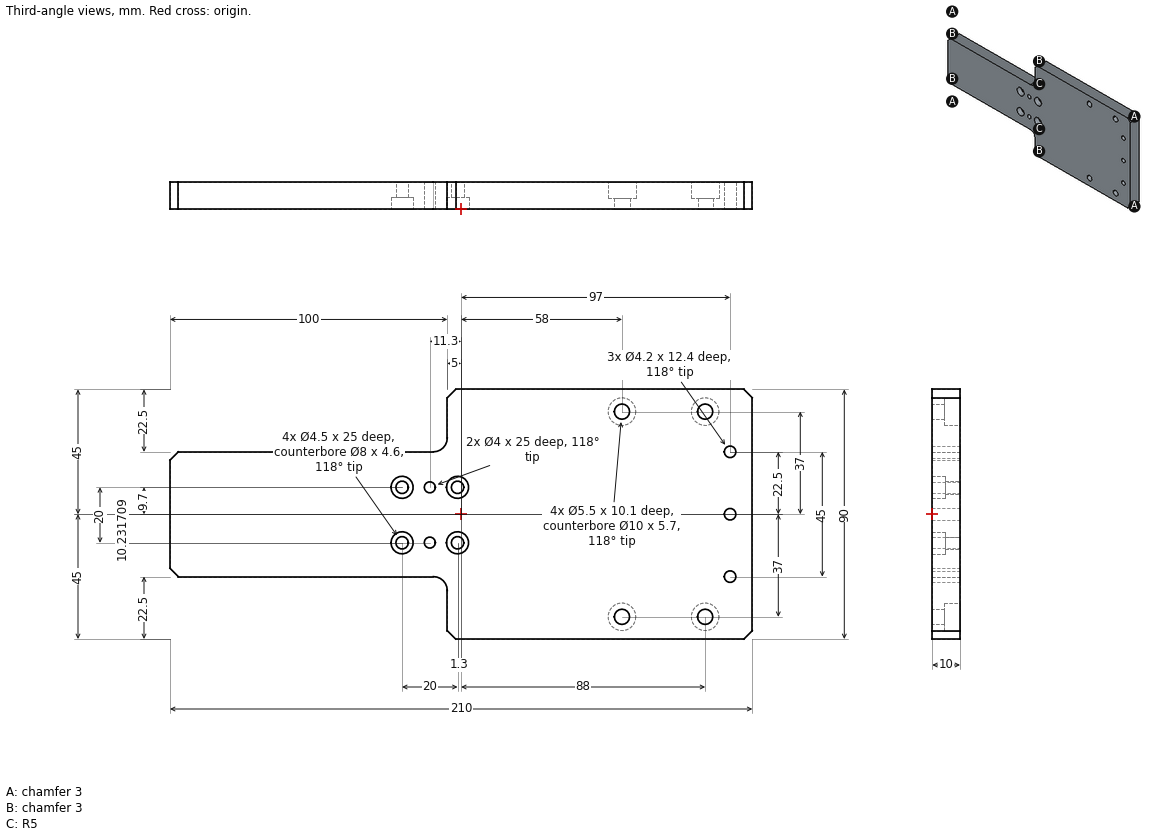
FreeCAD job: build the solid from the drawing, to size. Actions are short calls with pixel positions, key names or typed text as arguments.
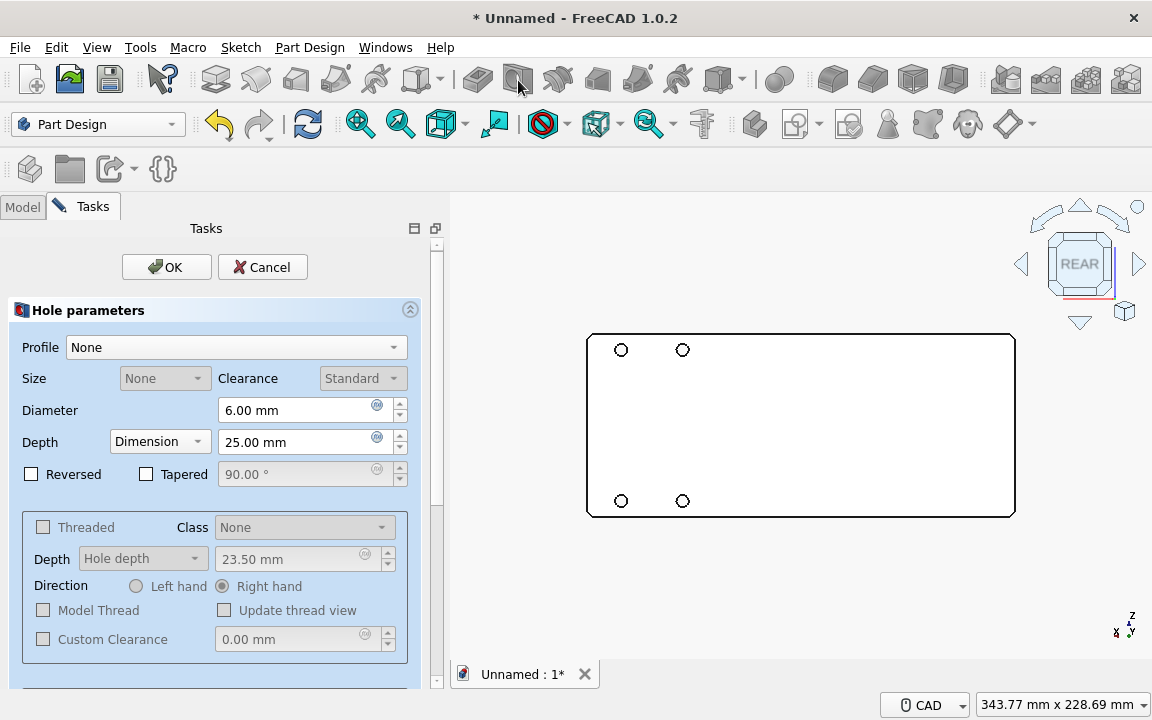
triple_click(305, 410)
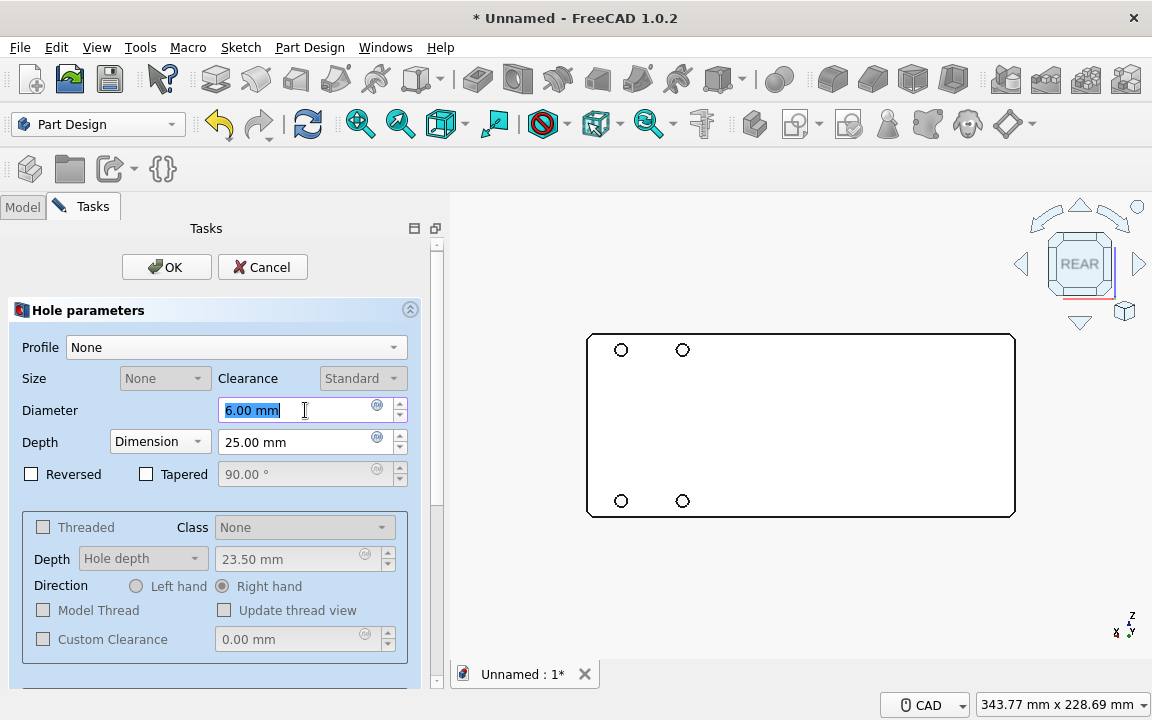
text(5.5)
key(Tab)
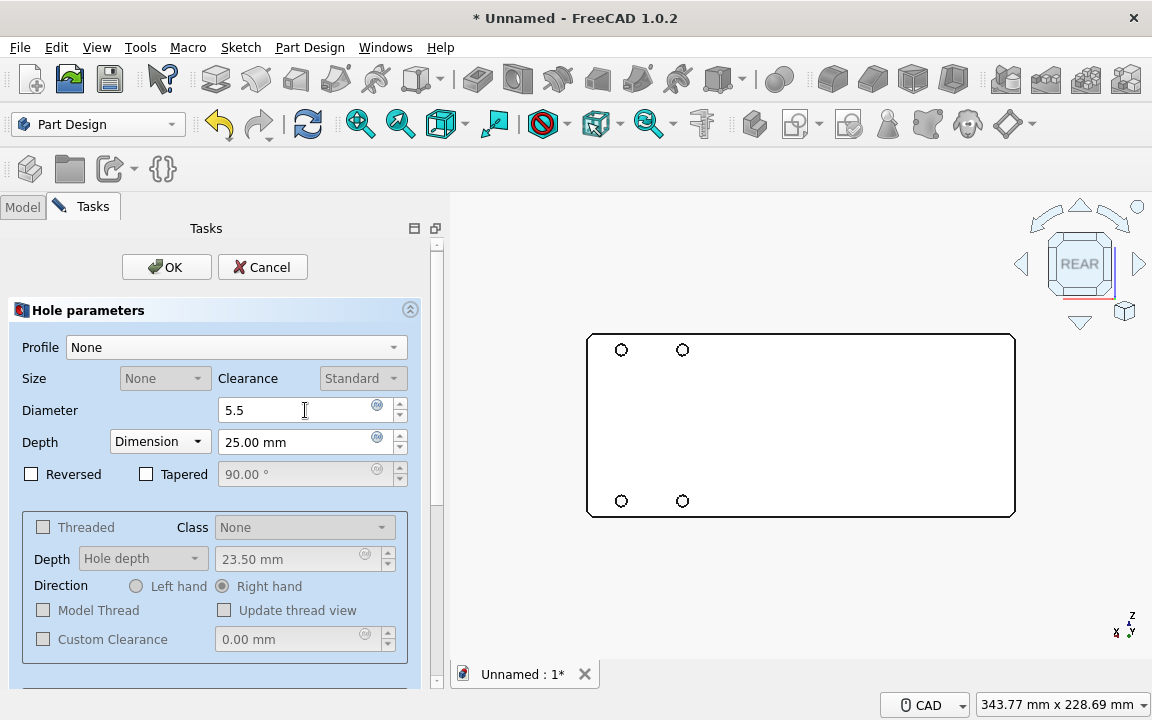
triple_click(305, 442)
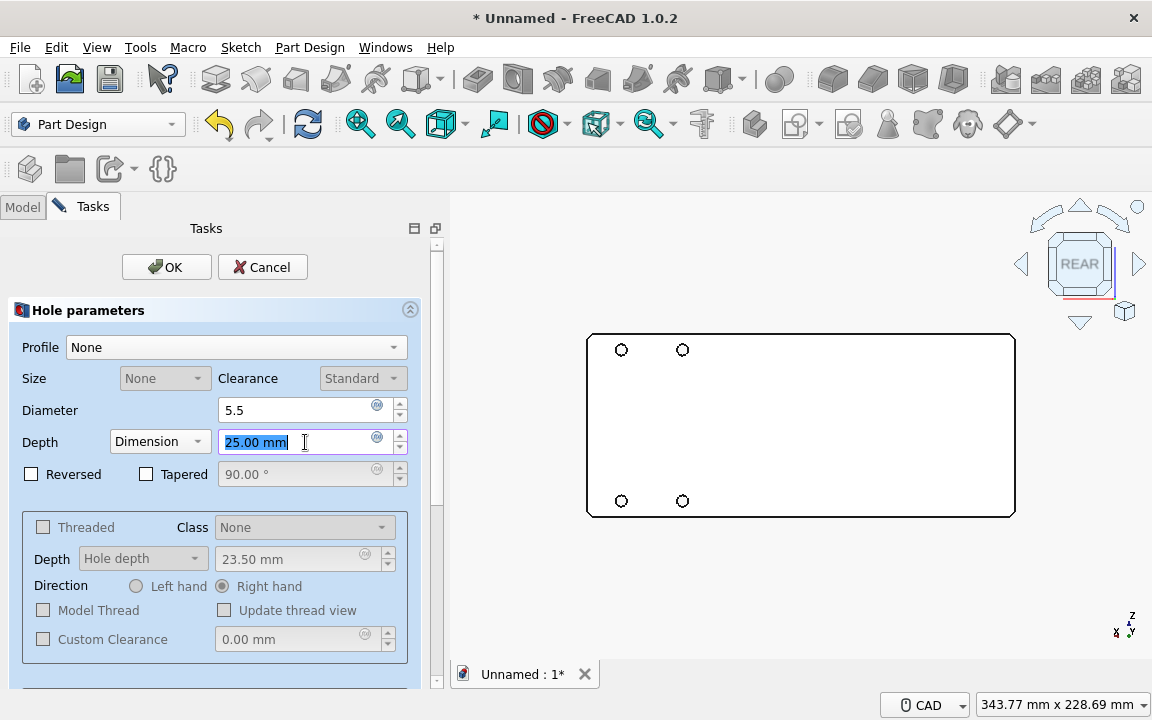
text(10.1)
key(Tab)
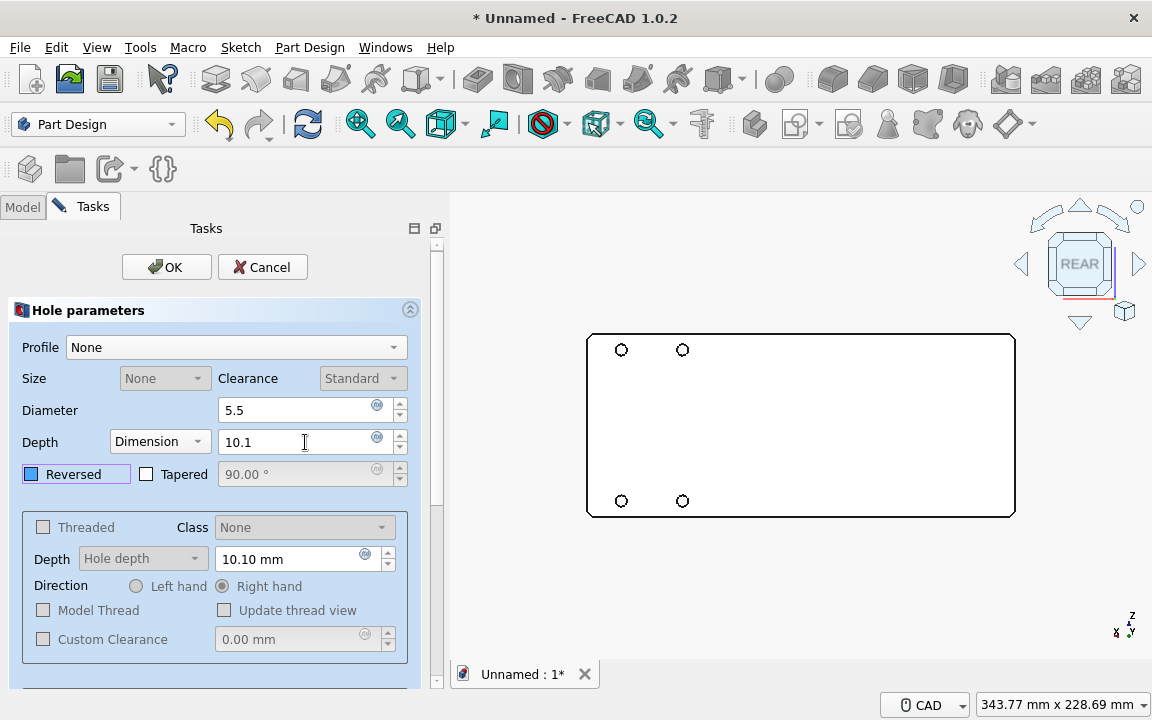
scroll(437, 463, down, 2)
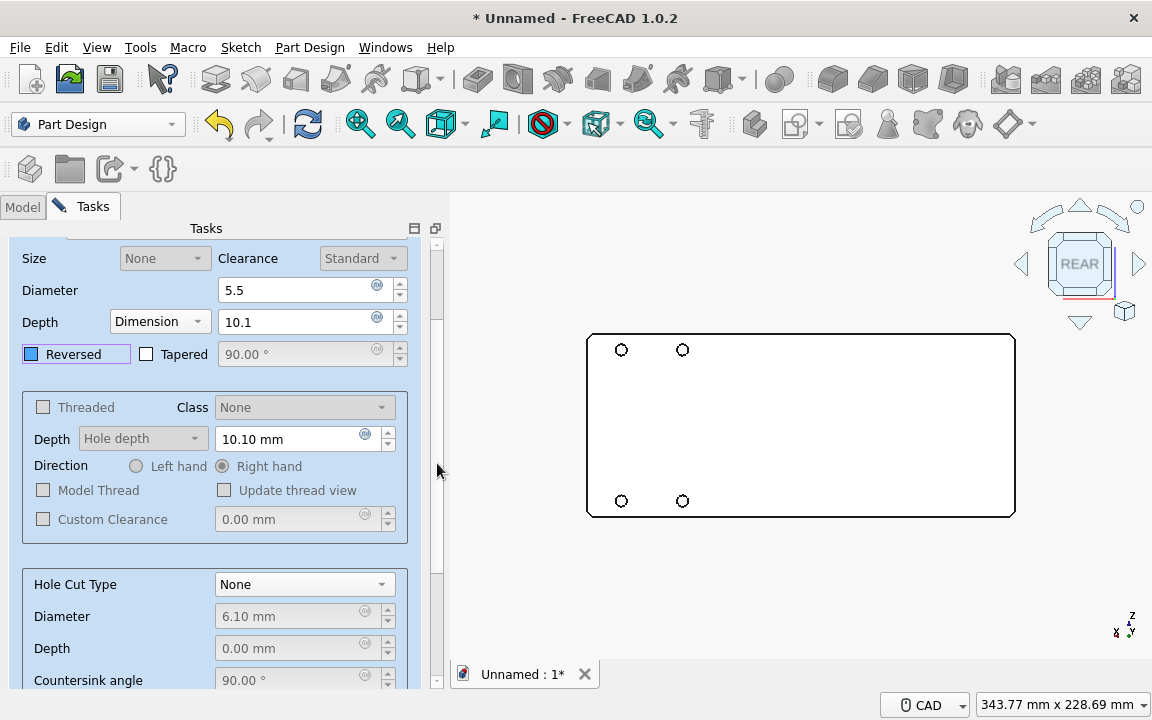
click(306, 584)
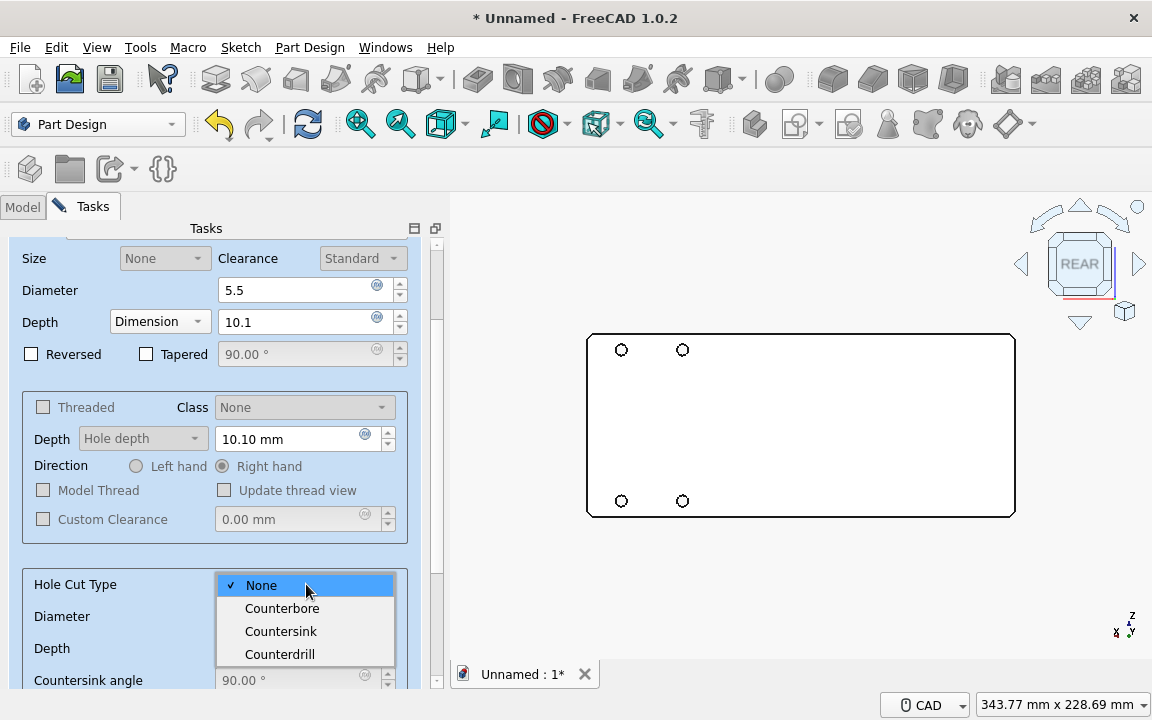
click(304, 608)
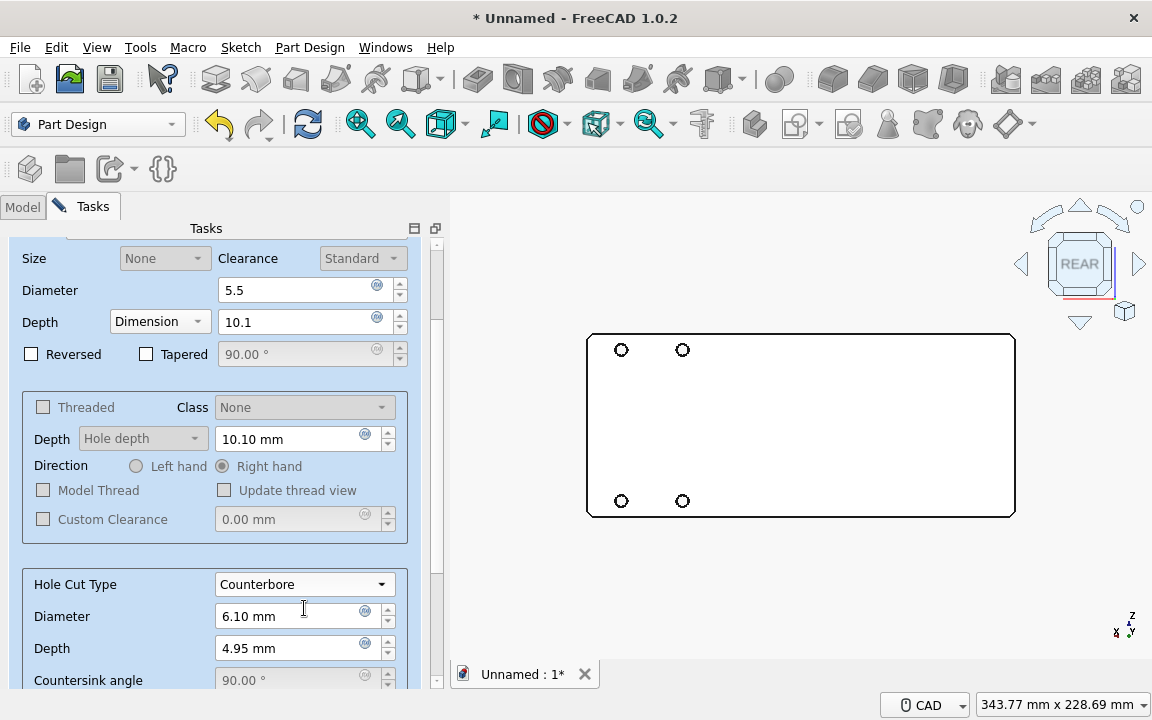
triple_click(298, 616)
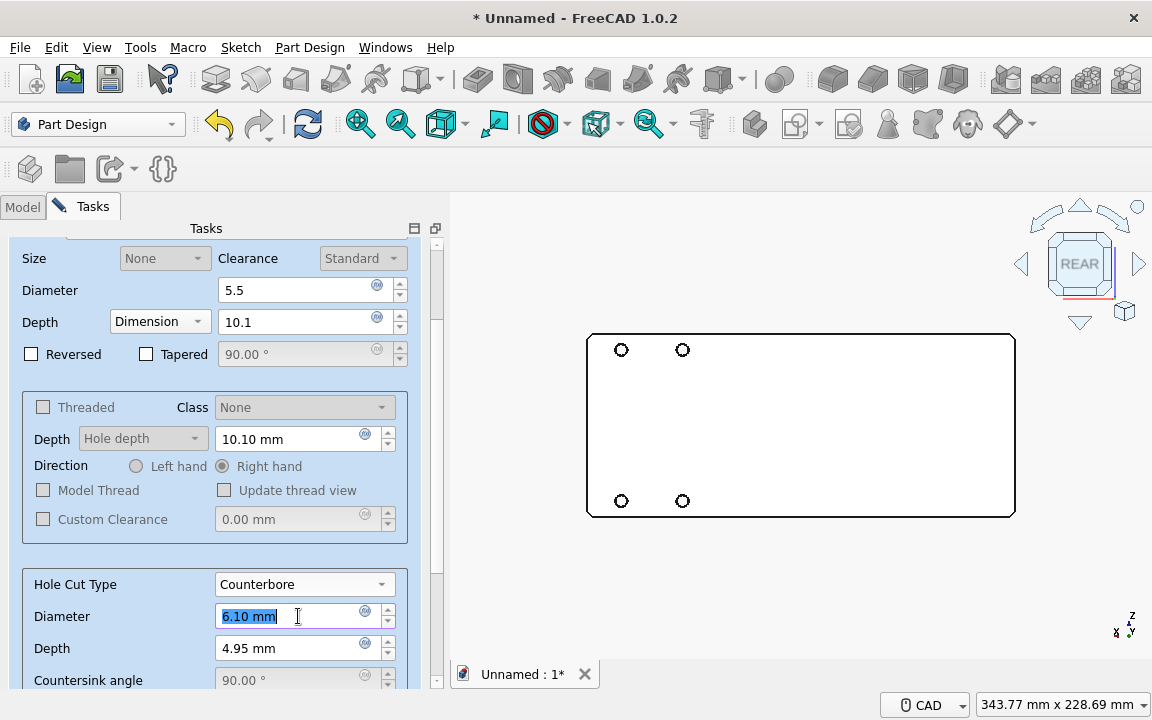
text(10)
key(Tab)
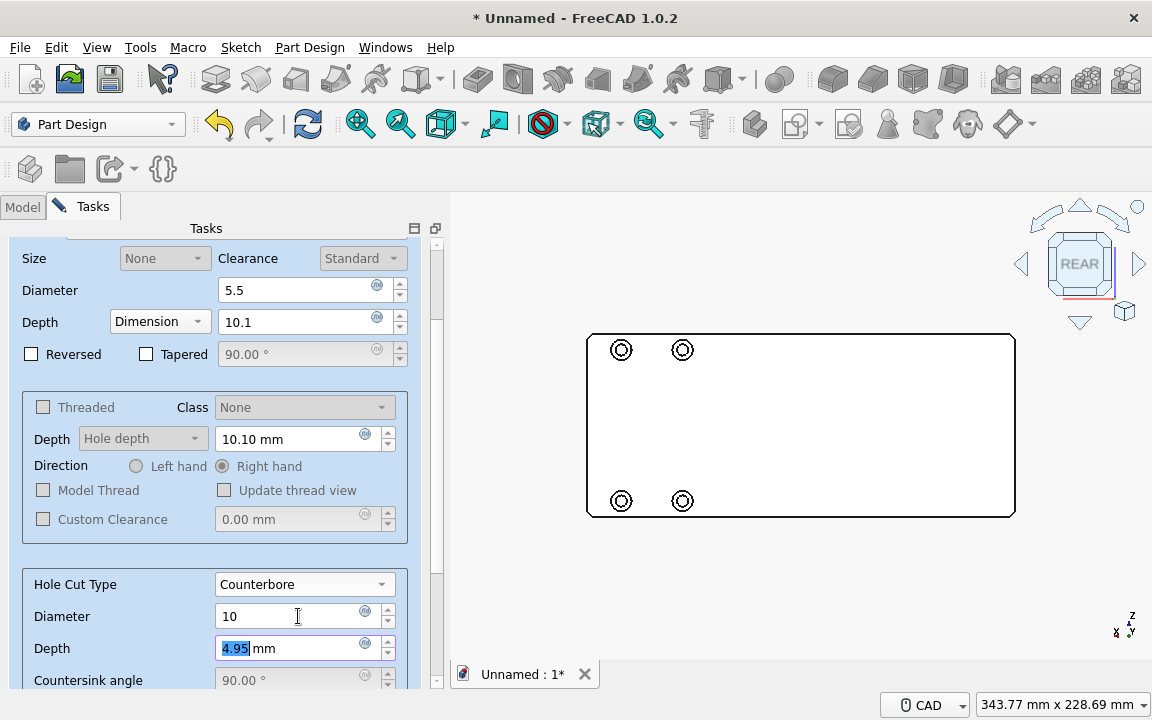
text(5.7)
key(Tab)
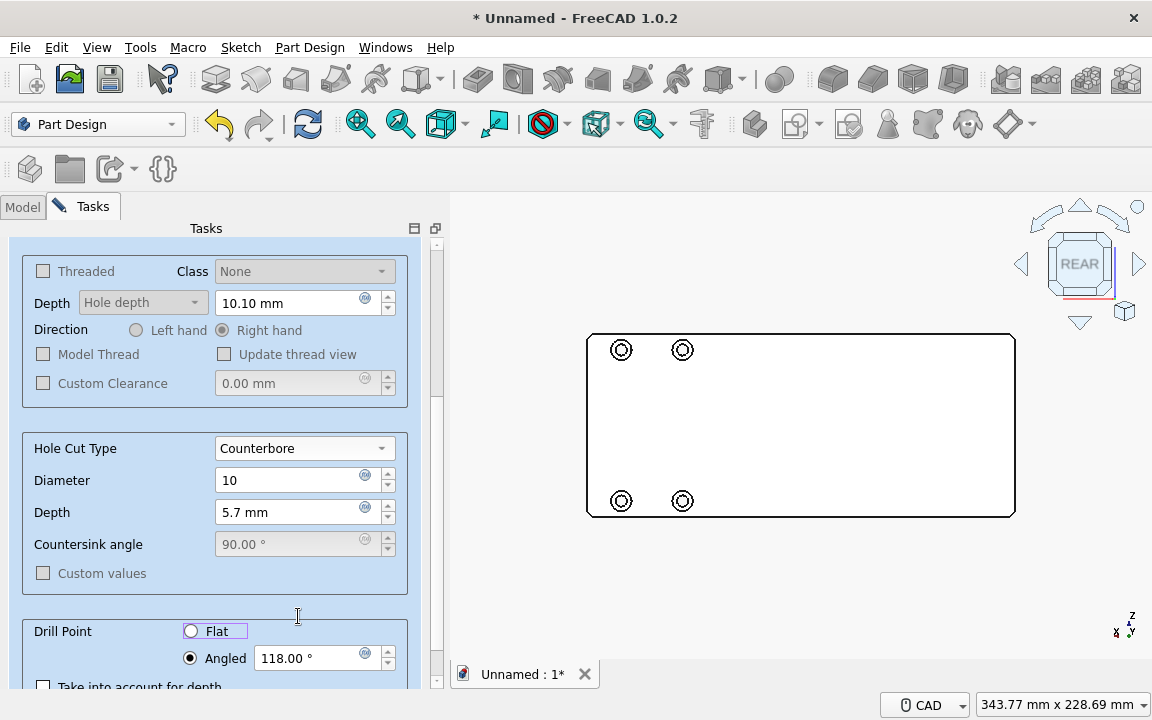
scroll(437, 463, up, 6)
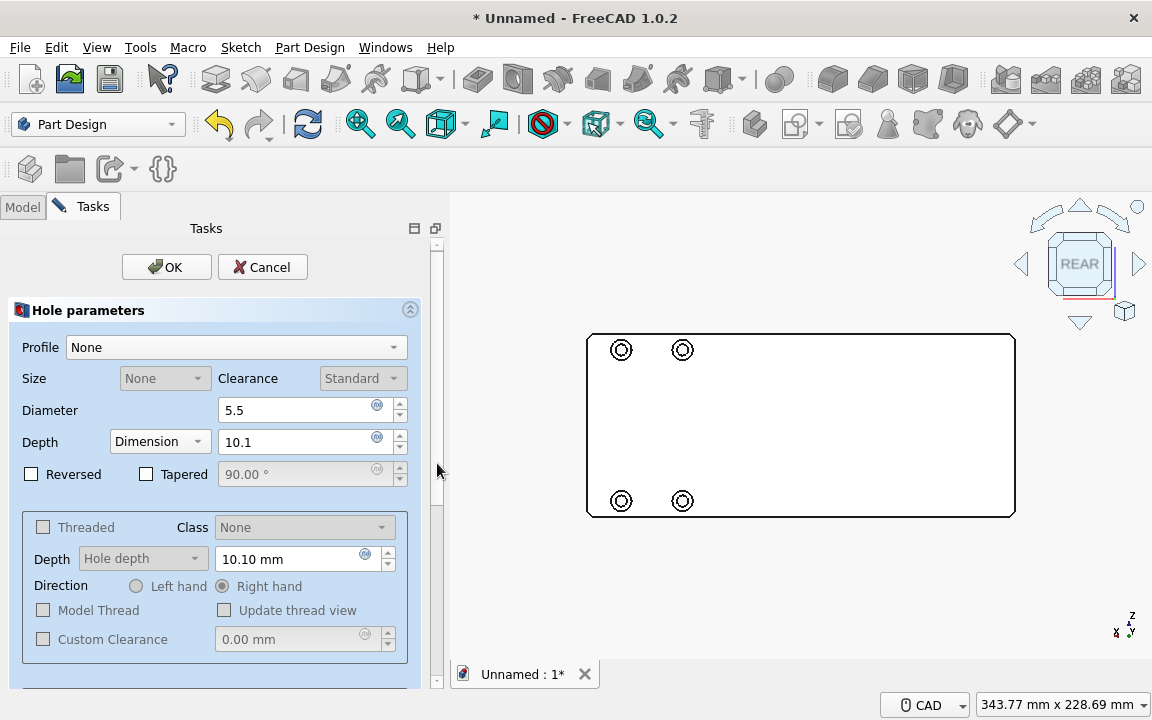
click(167, 267)